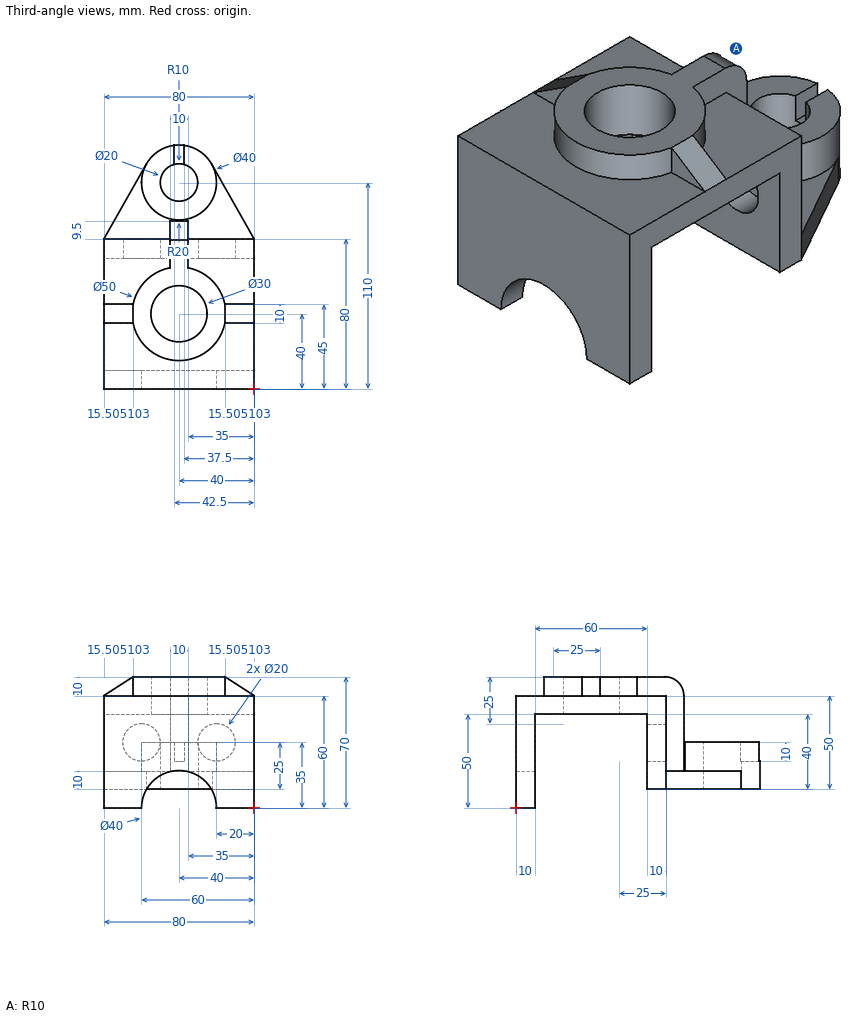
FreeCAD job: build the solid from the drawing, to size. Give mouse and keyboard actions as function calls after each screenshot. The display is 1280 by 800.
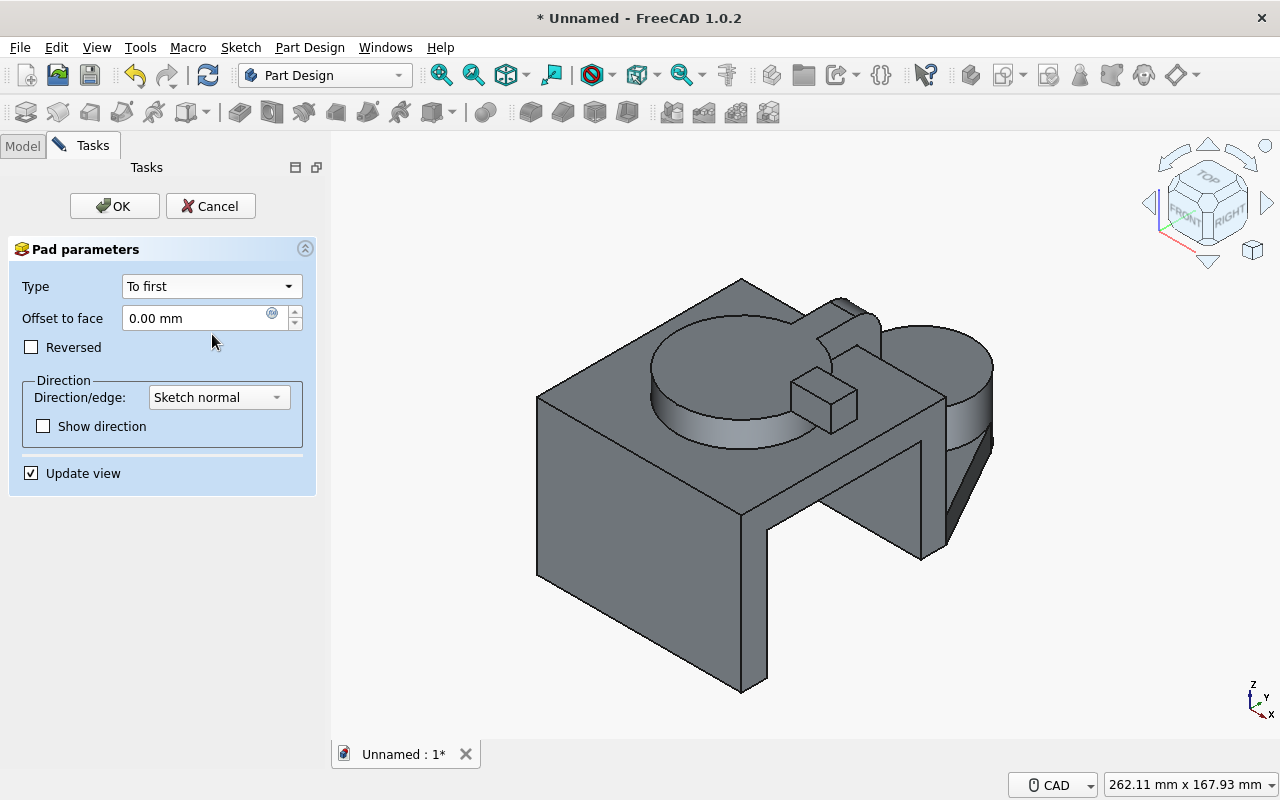
click(30, 347)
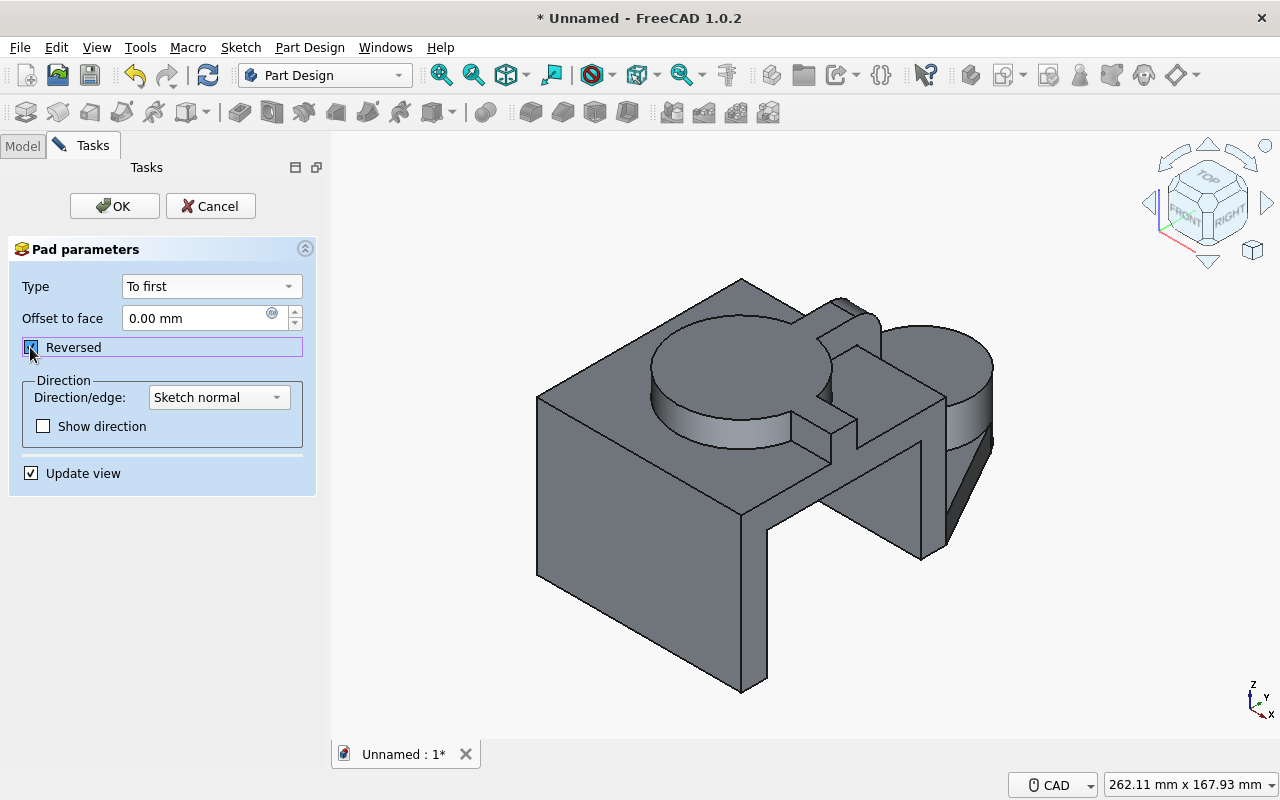
click(115, 206)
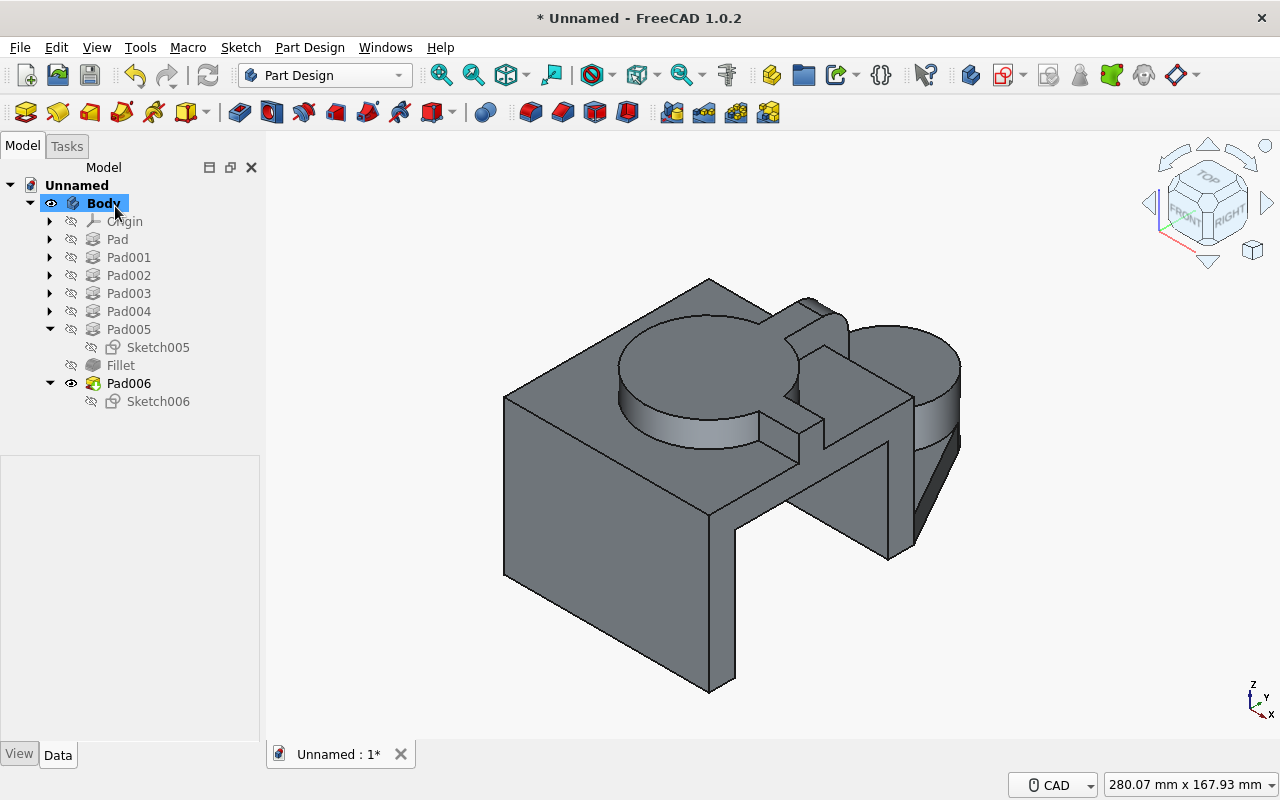
click(699, 367)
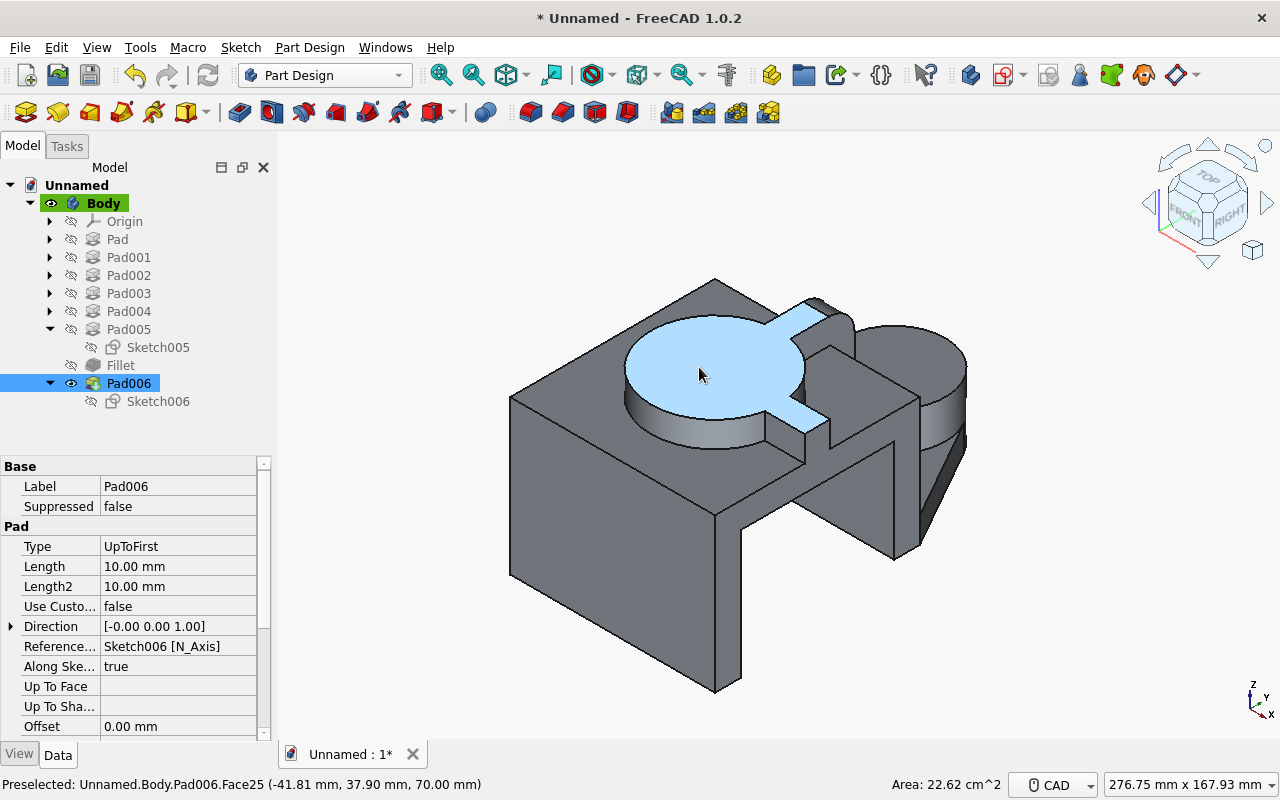
click(1004, 76)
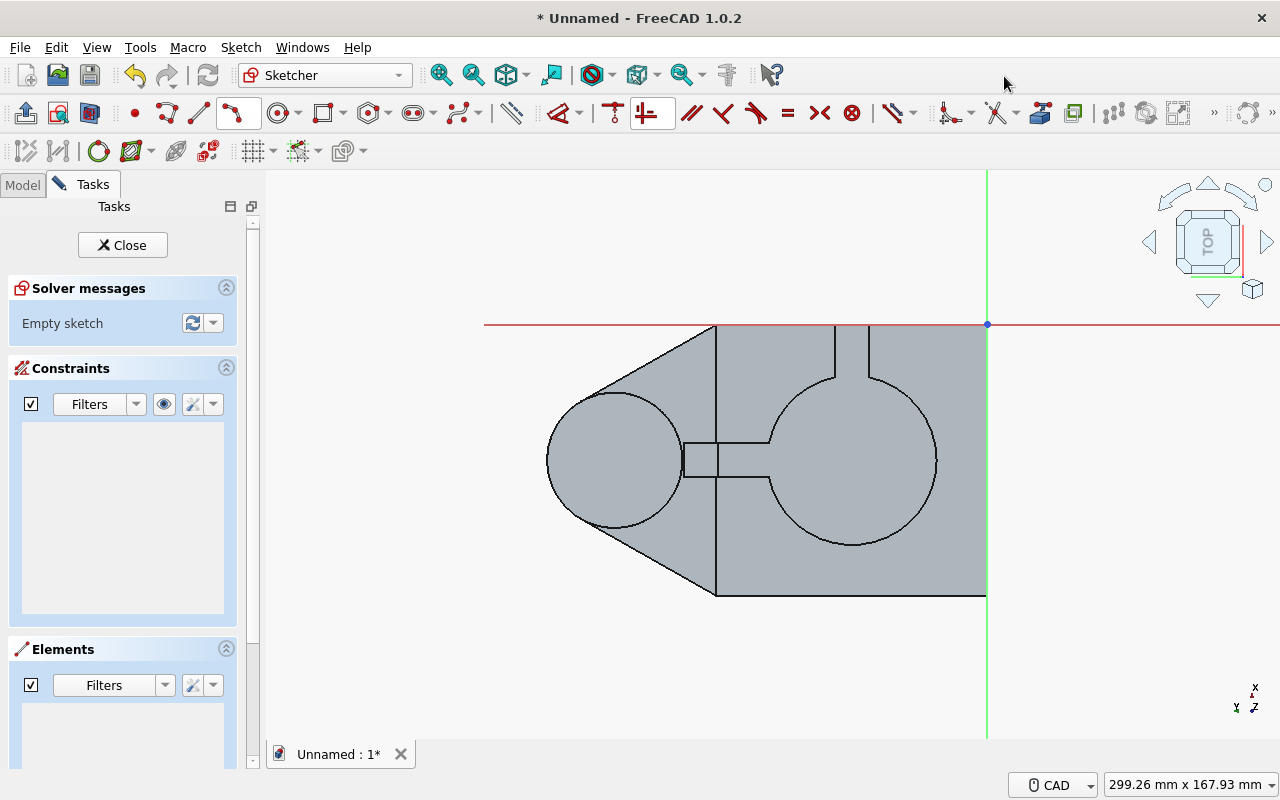
scroll(875, 588, up, 10)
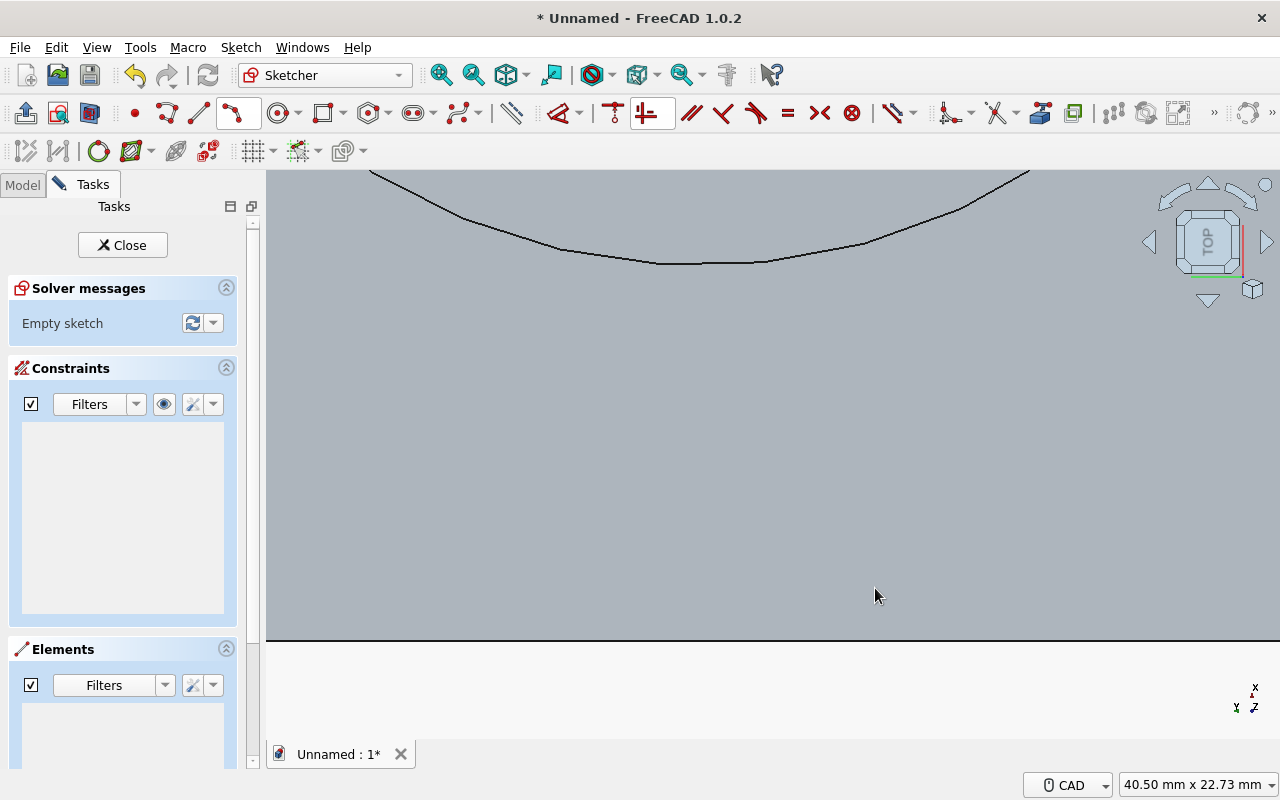
click(324, 114)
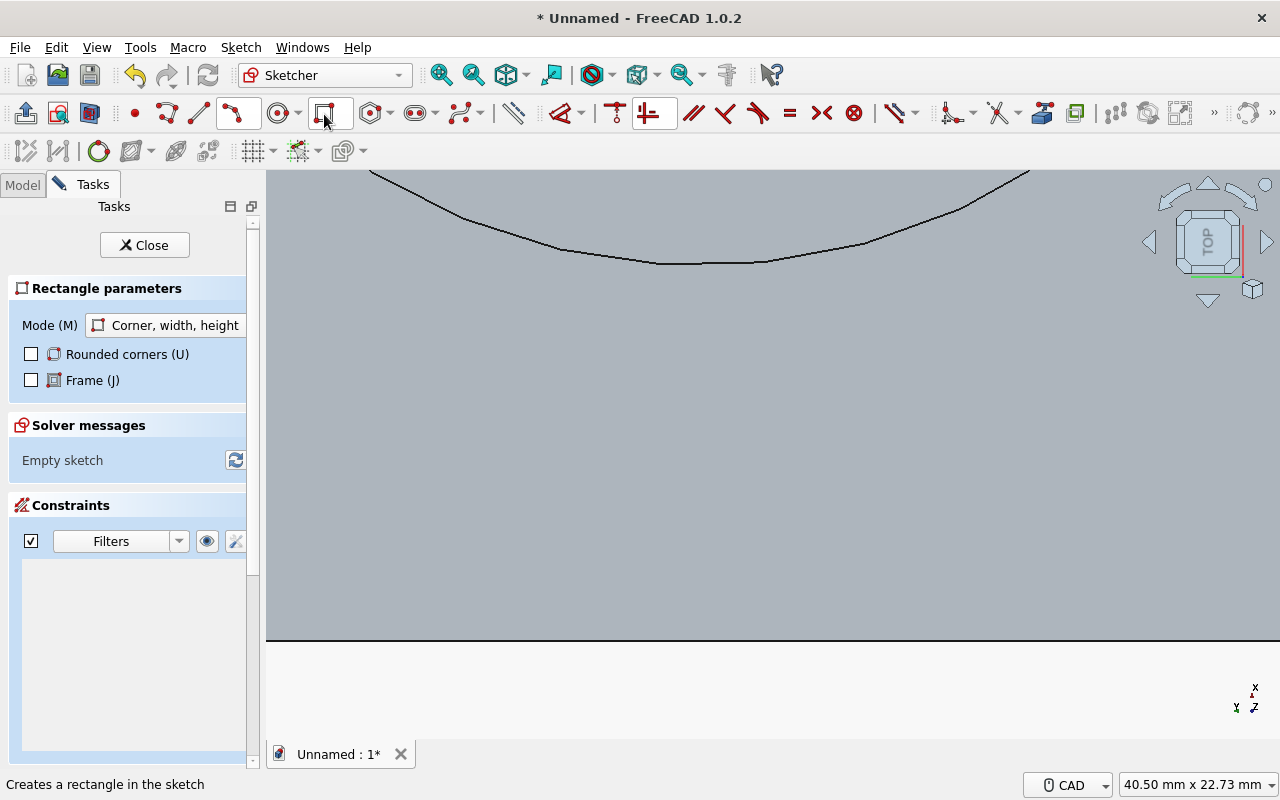
click(575, 253)
move(826, 641)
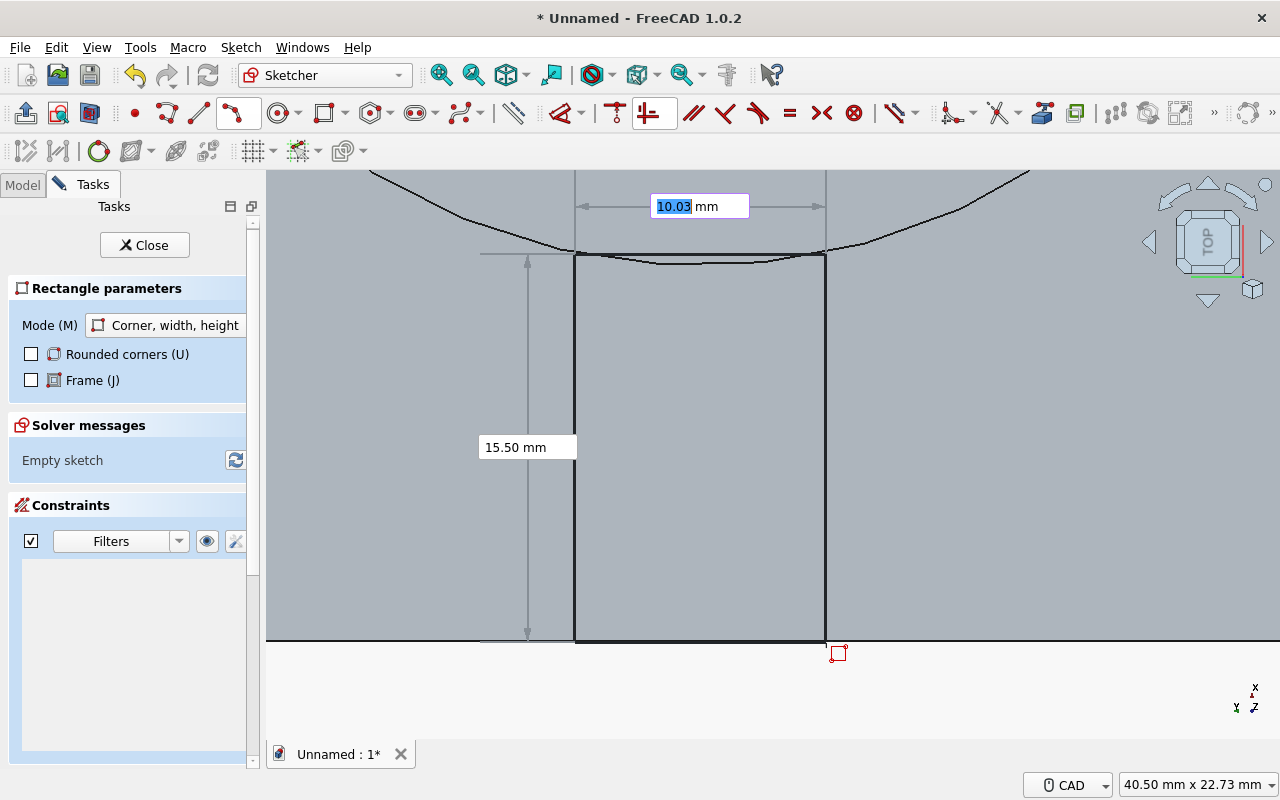
text(10)
key(Tab)
text(15.505103)
key(Return)
key(Escape)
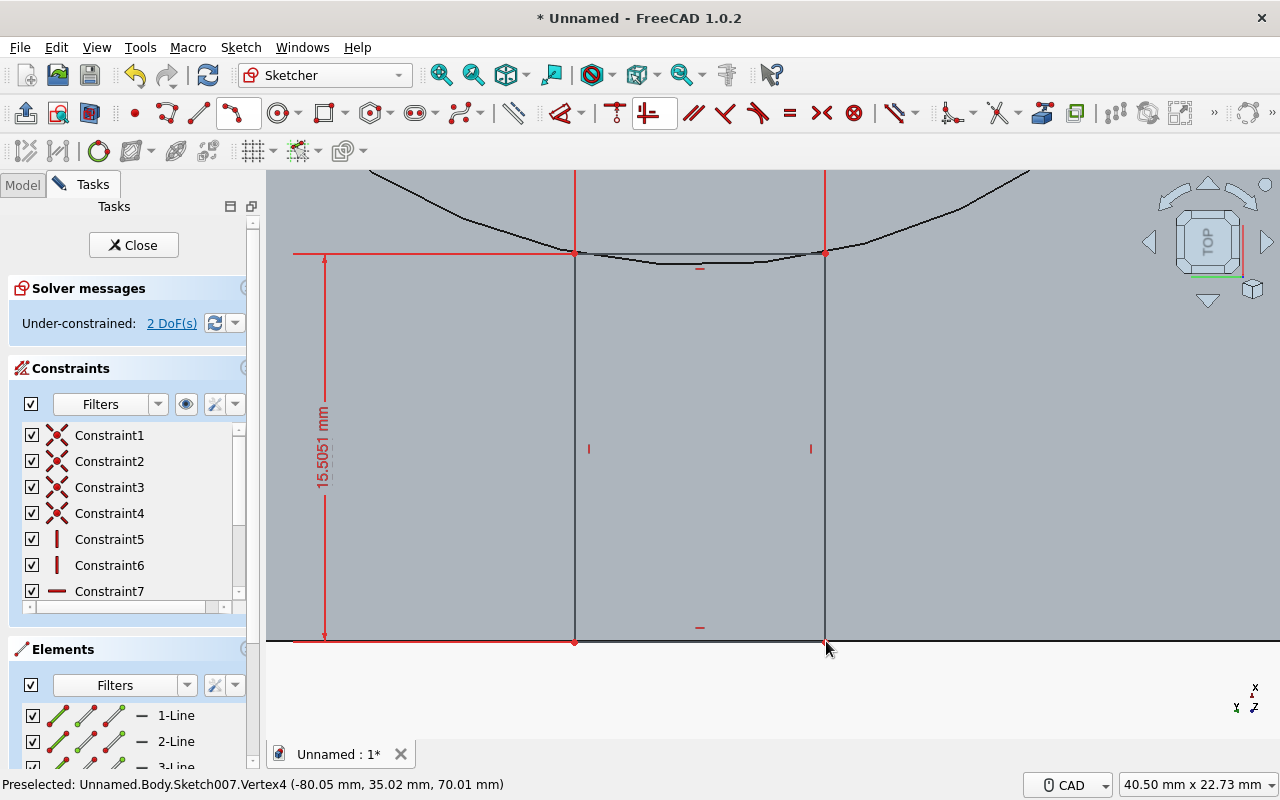
click(560, 114)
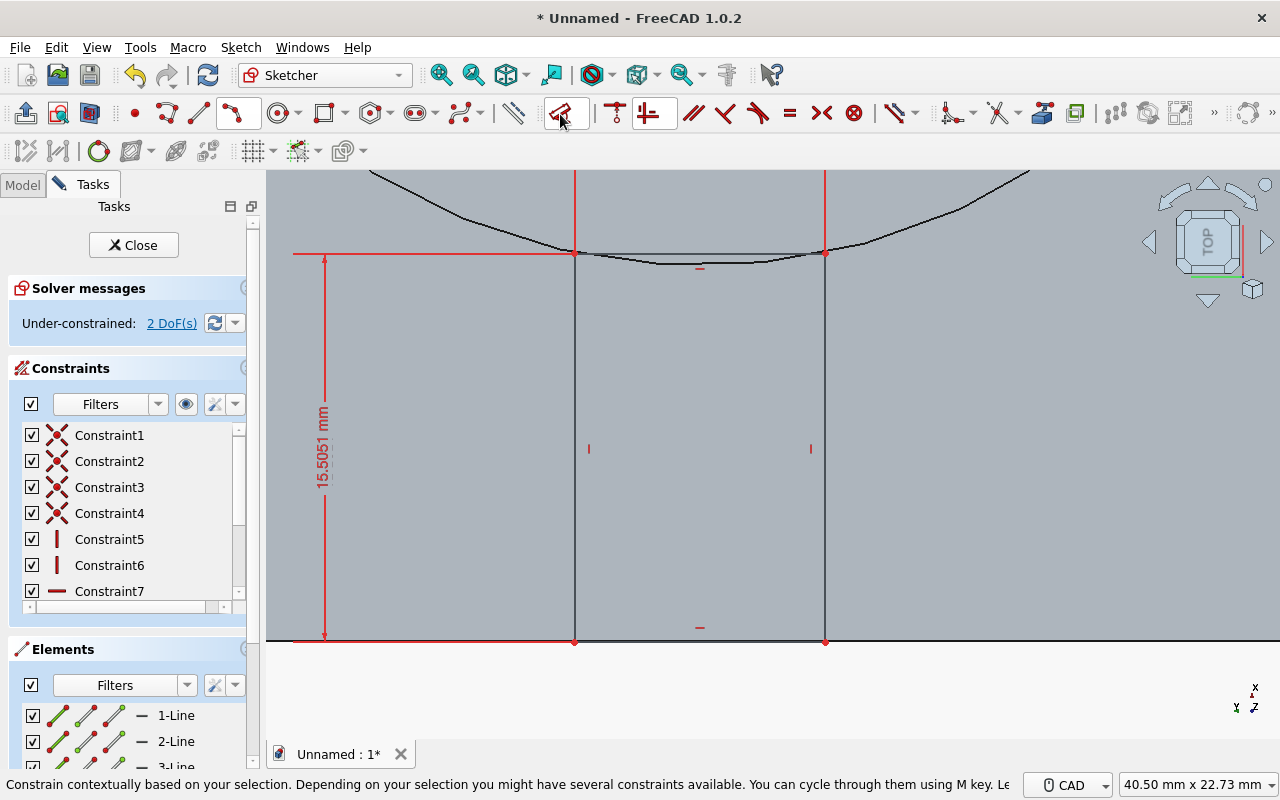
click(575, 254)
click(845, 288)